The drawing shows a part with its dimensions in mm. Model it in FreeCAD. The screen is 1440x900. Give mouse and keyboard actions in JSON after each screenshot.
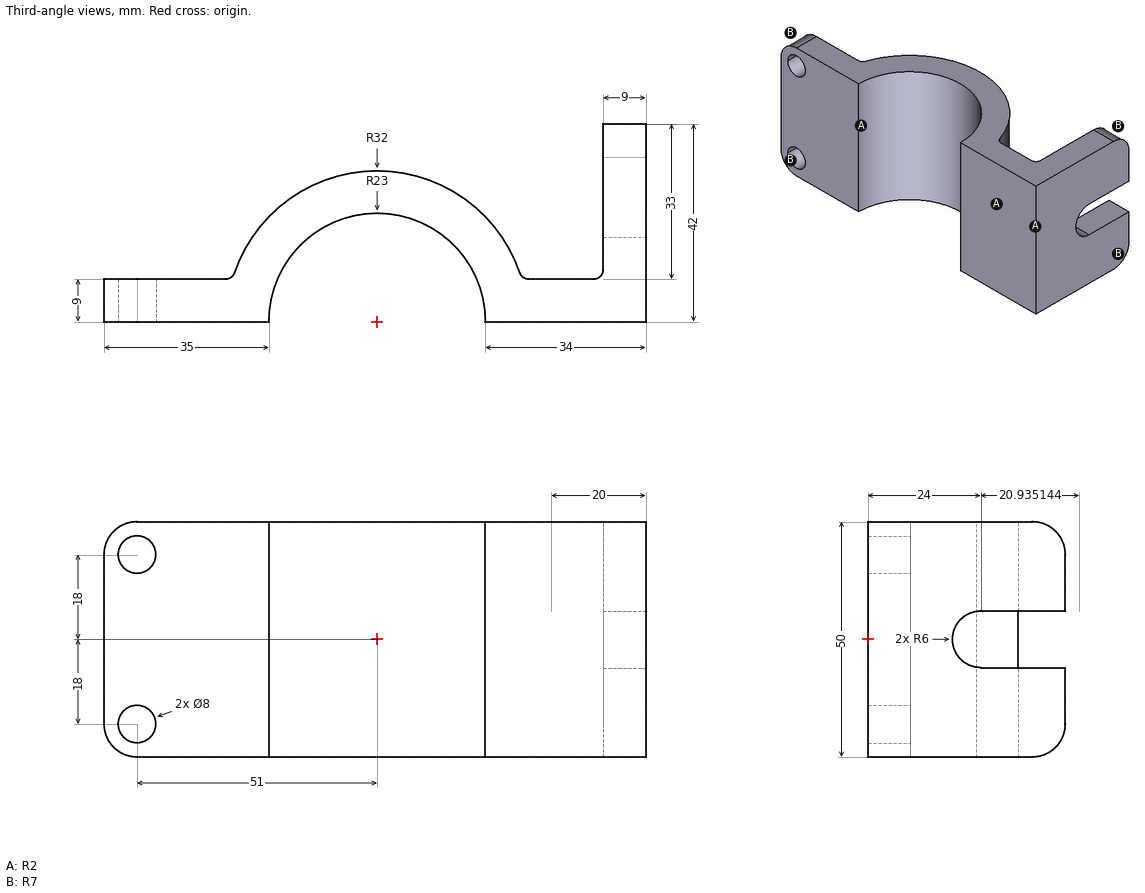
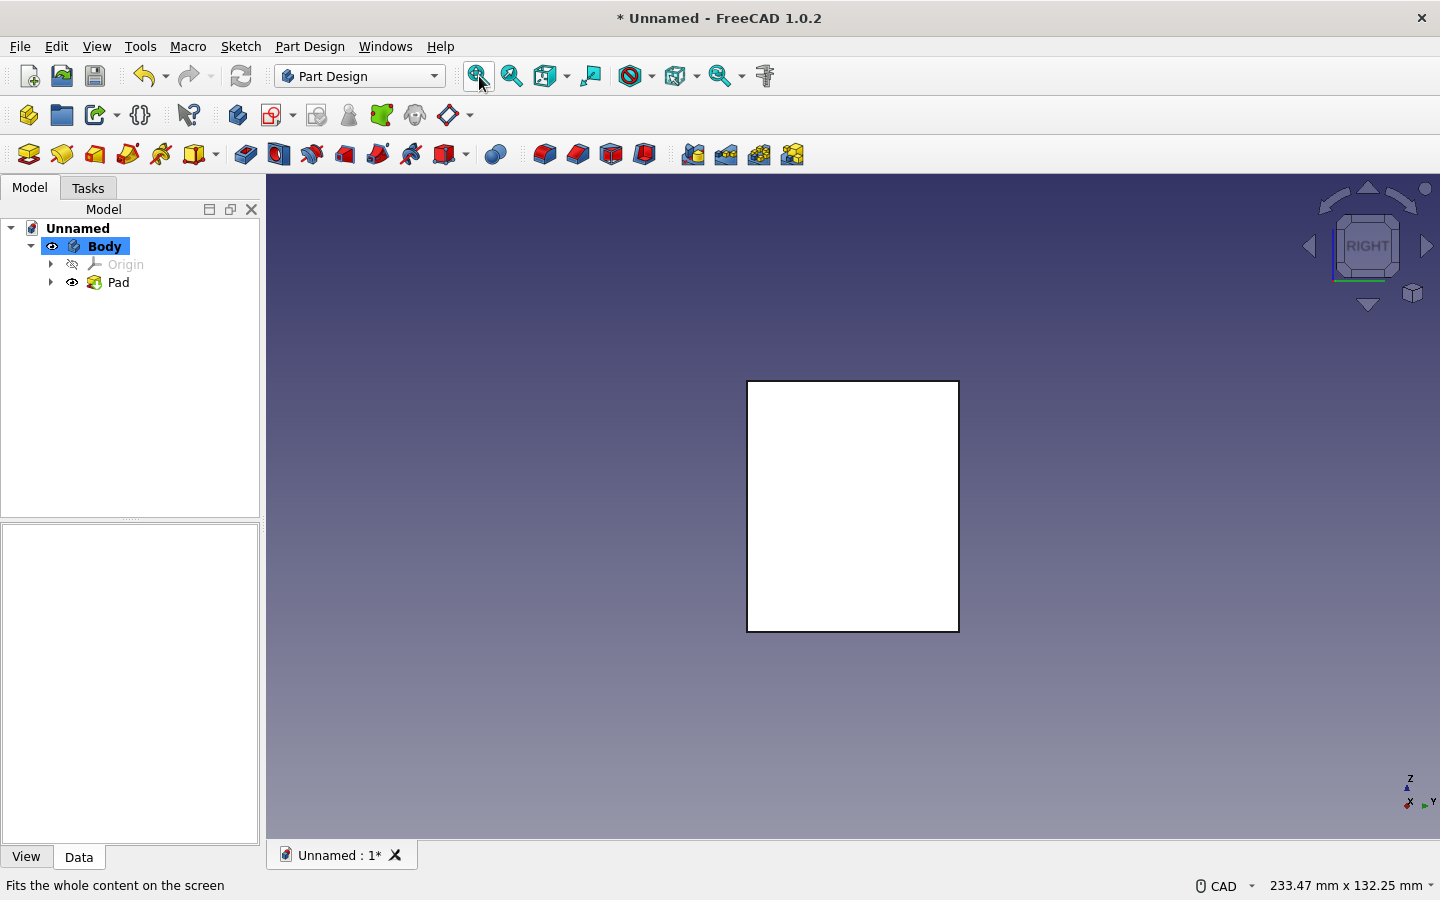
{"action": "key", "text": "5"}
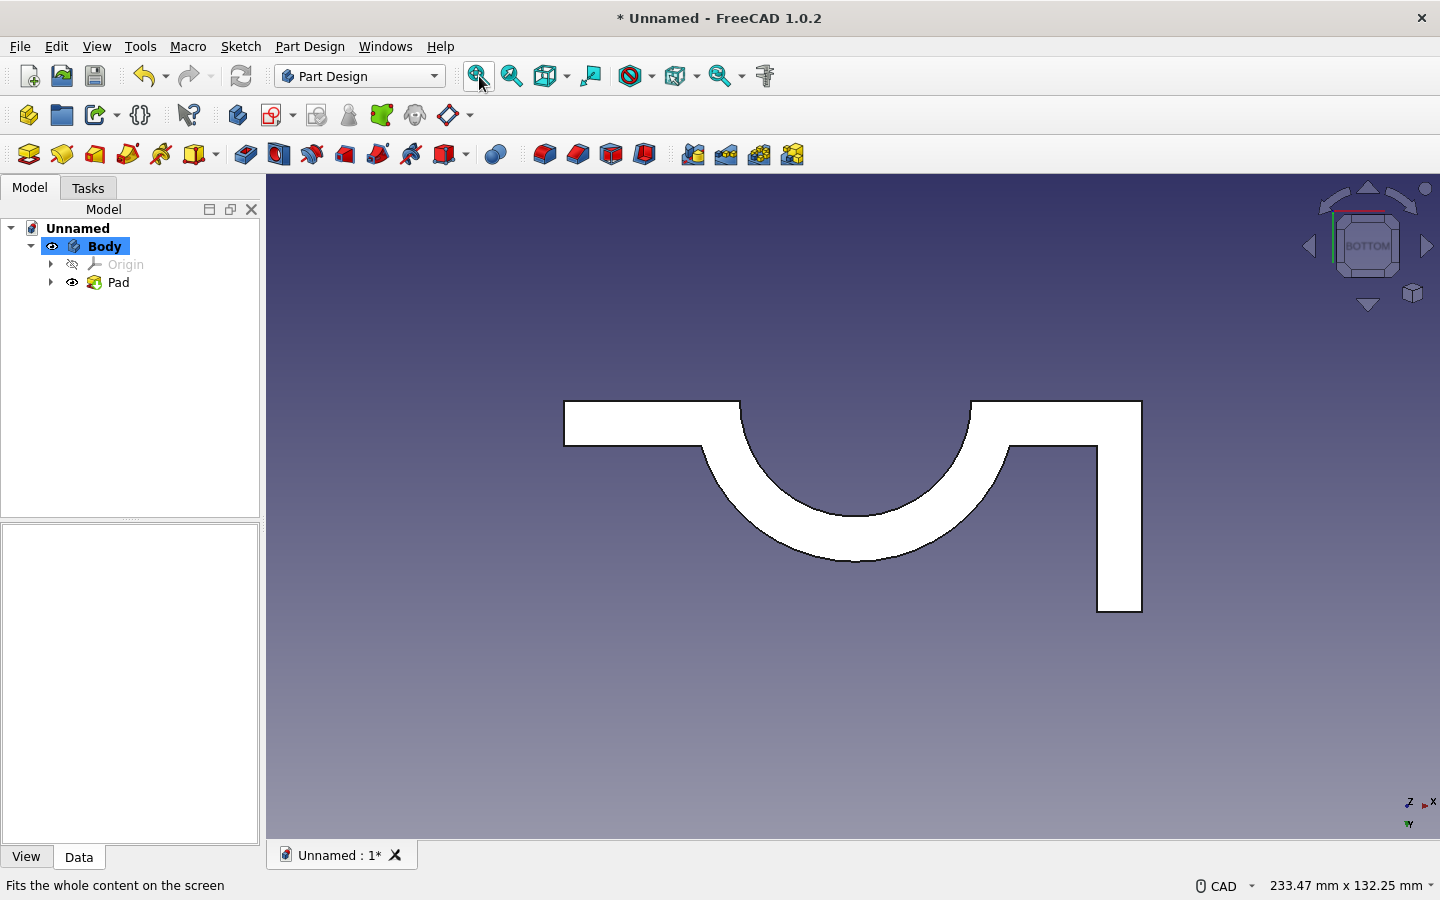
{"action": "key", "text": "4"}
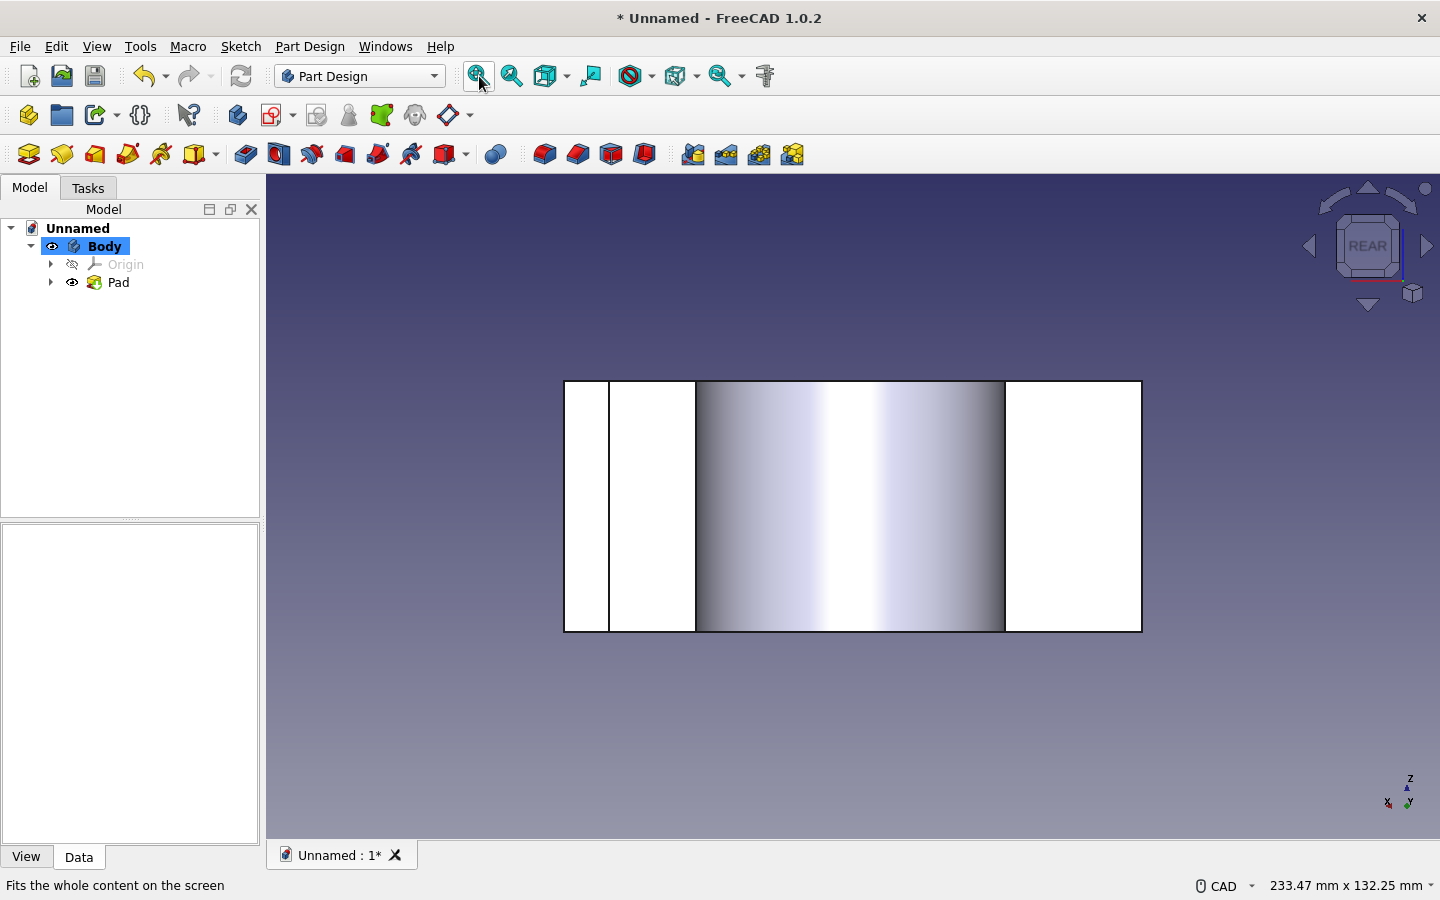
{"action": "key", "text": "6"}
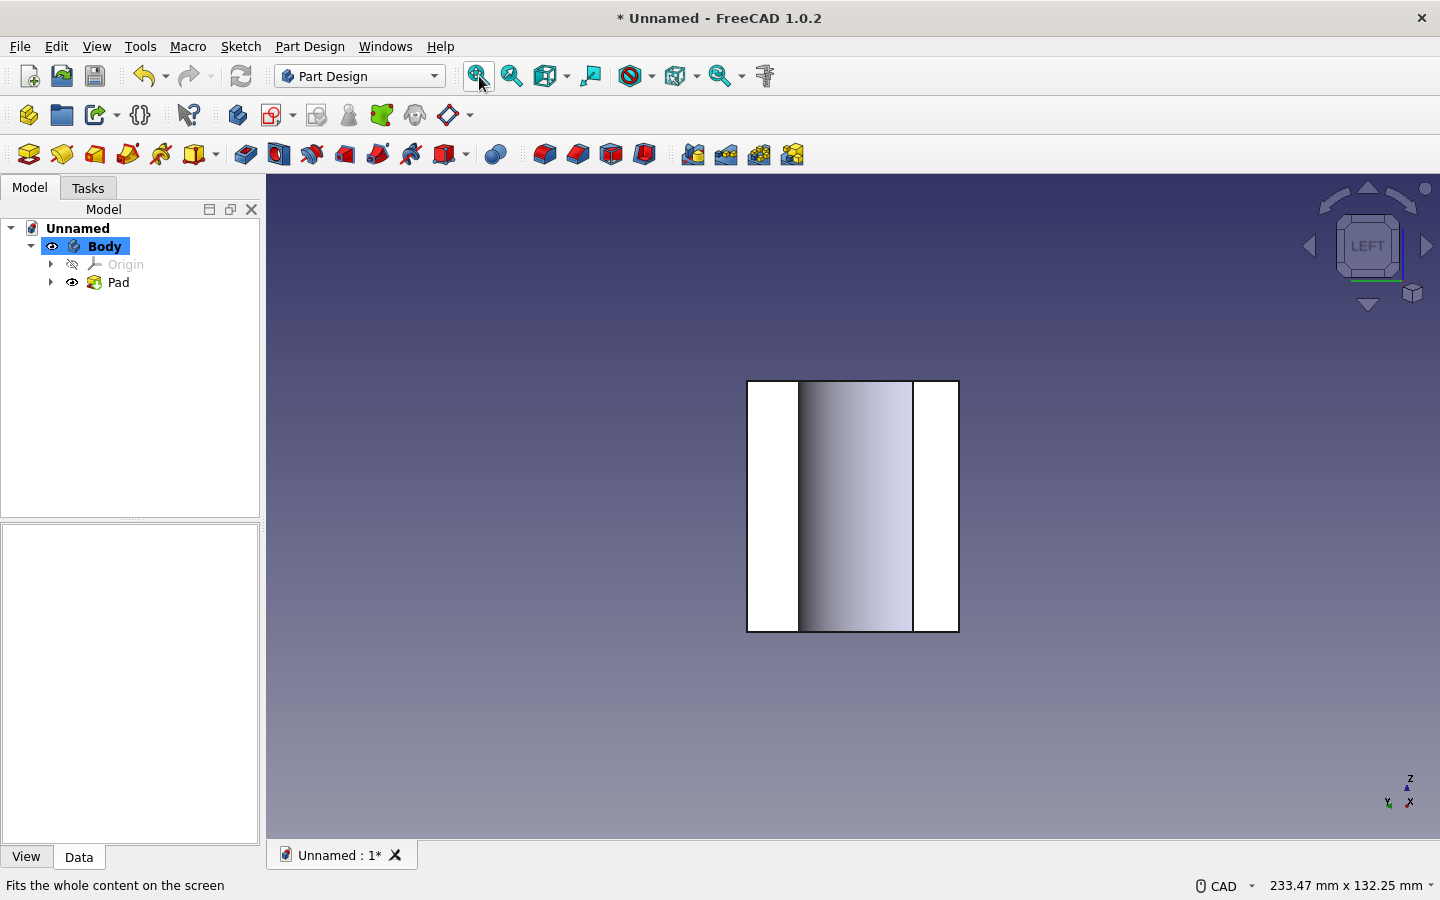
{"action": "left_click", "coordinate": [479, 76]}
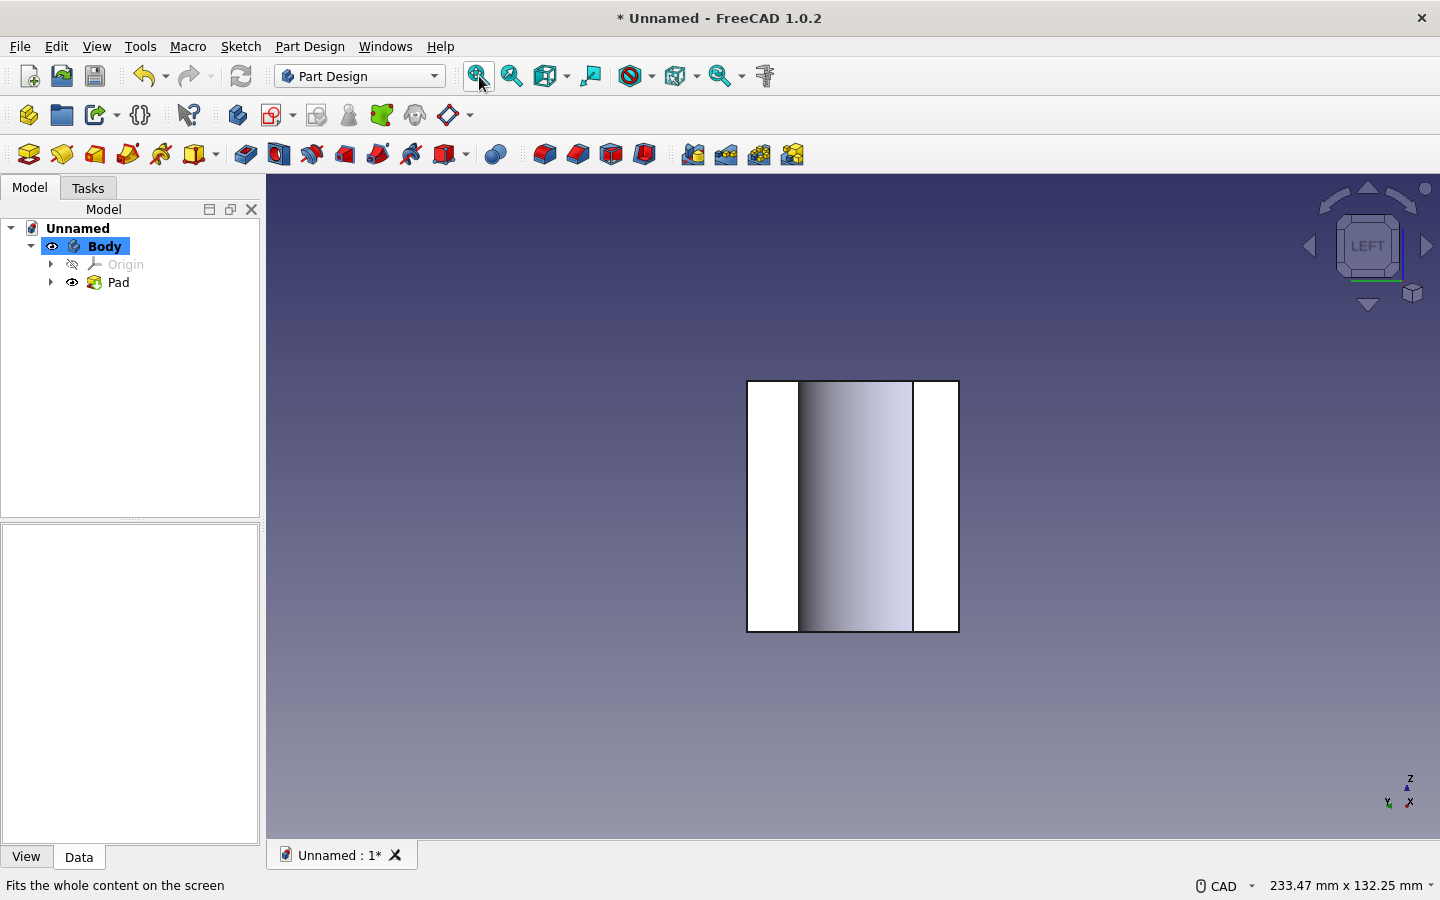
{"action": "key", "text": "v 3"}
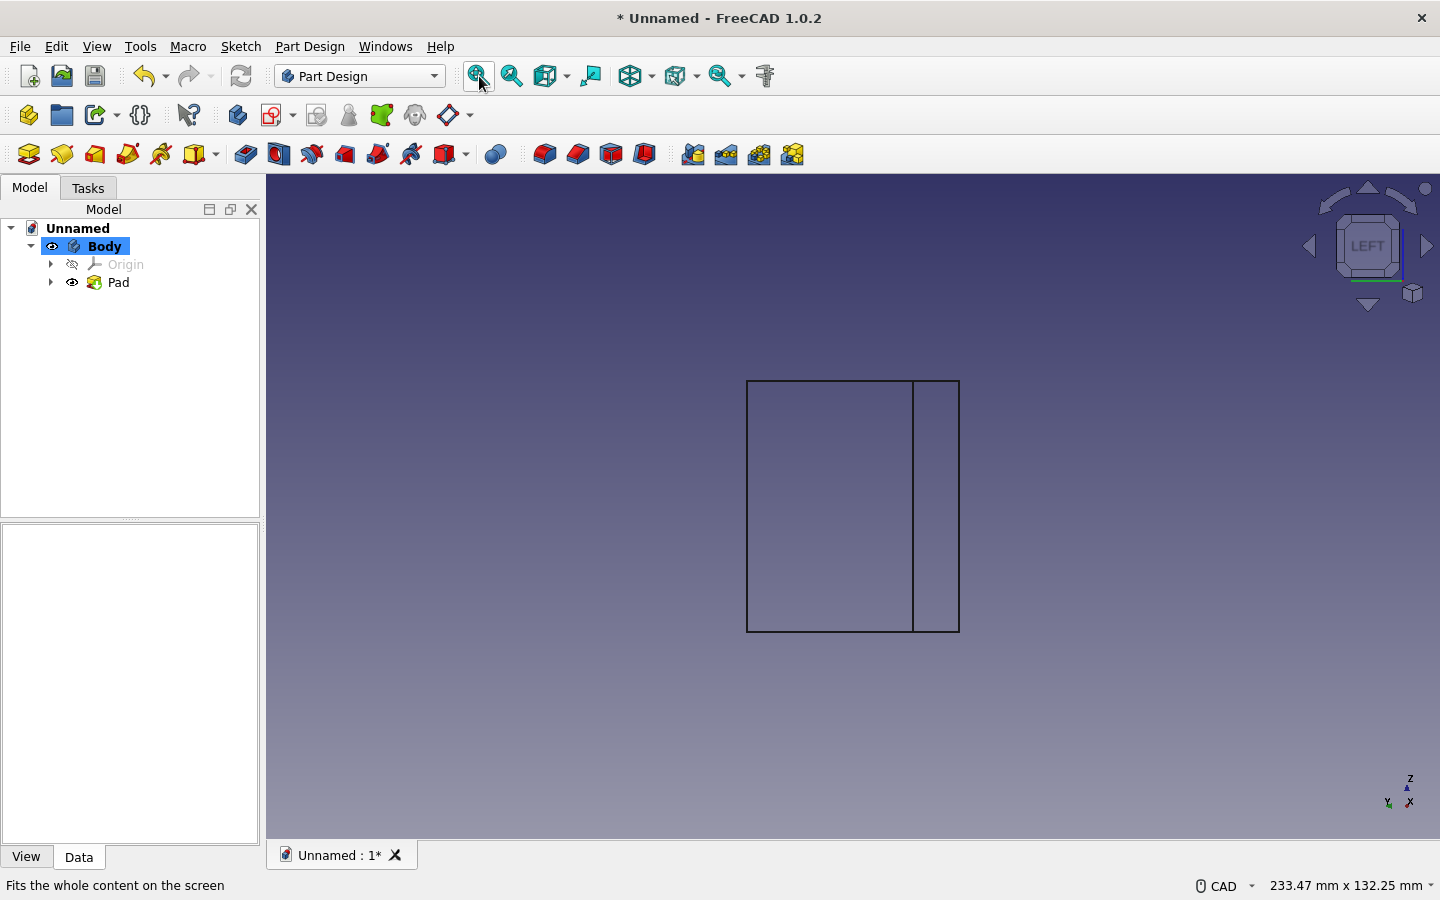
{"action": "key", "text": "0"}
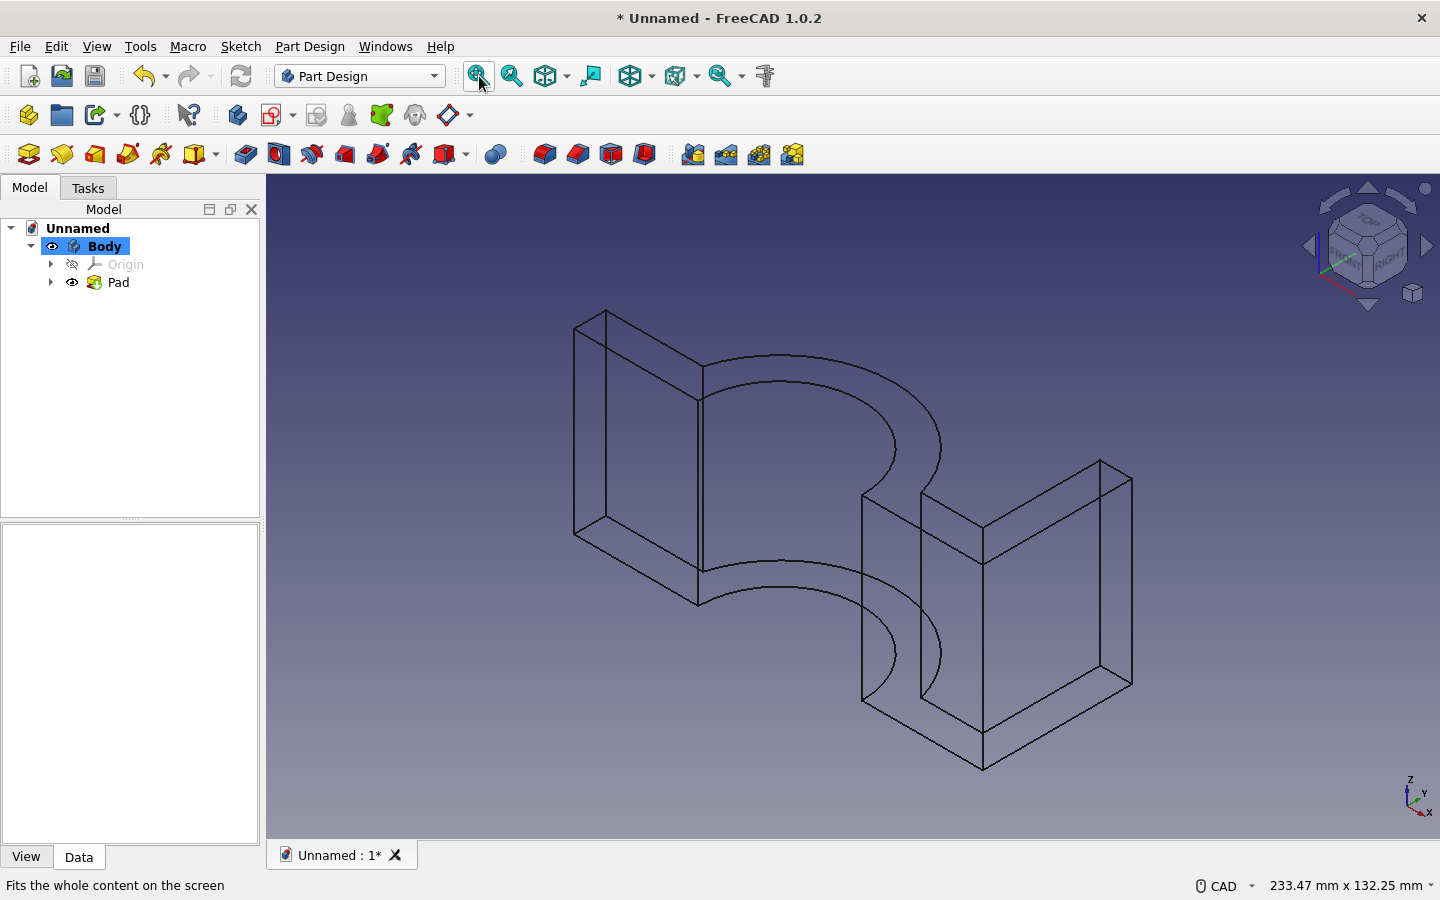
{"action": "left_click", "coordinate": [703, 390]}